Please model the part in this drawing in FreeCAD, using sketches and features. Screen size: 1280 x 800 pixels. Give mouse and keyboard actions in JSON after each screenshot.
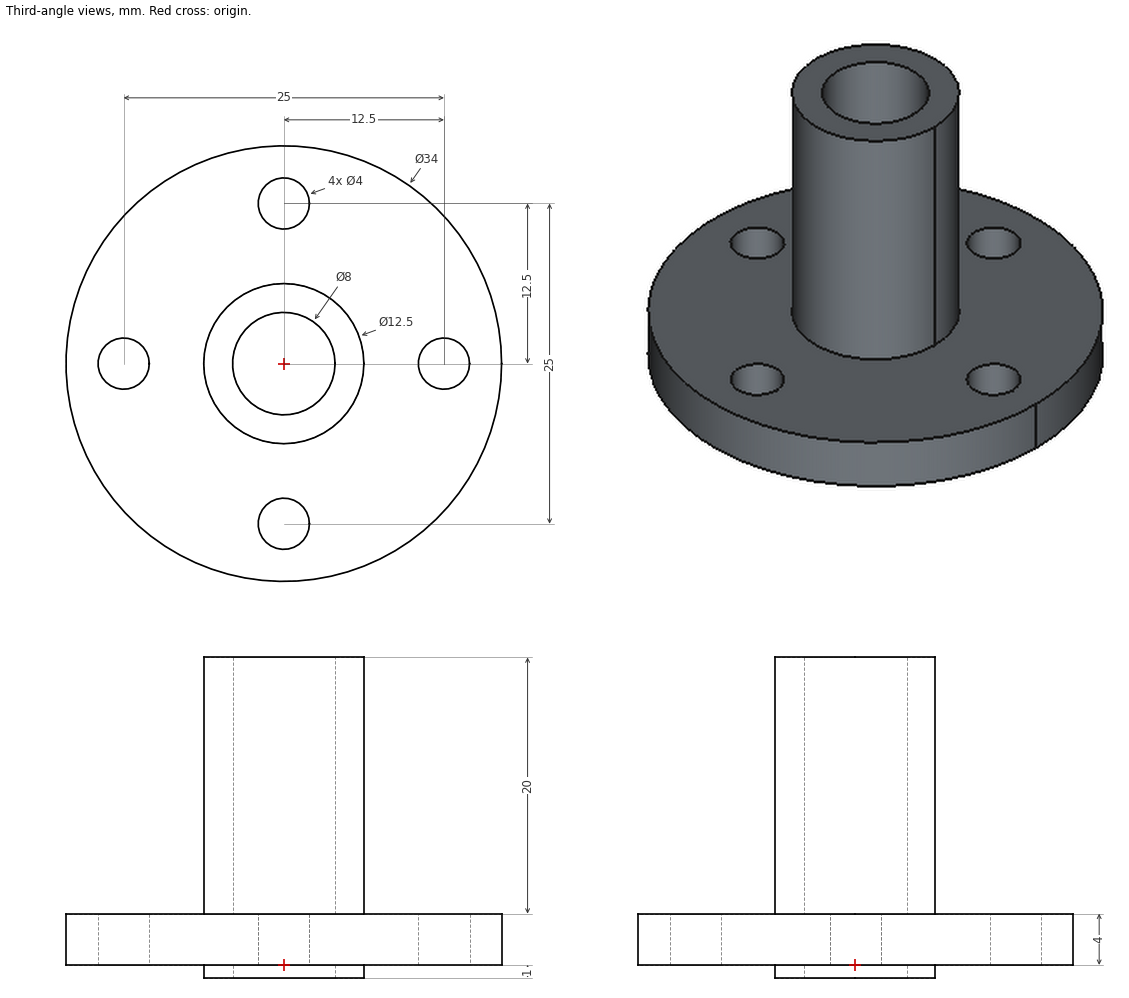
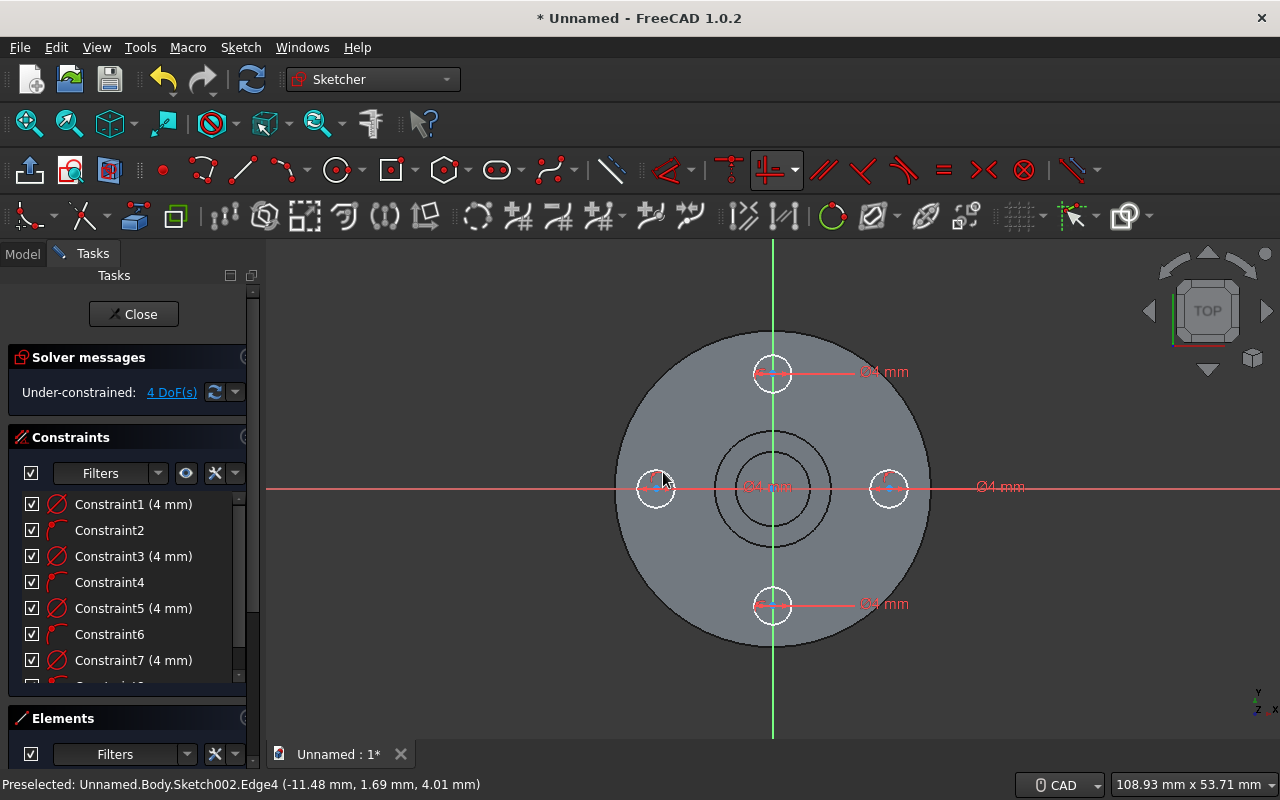
{"action": "left_click", "coordinate": [666, 170]}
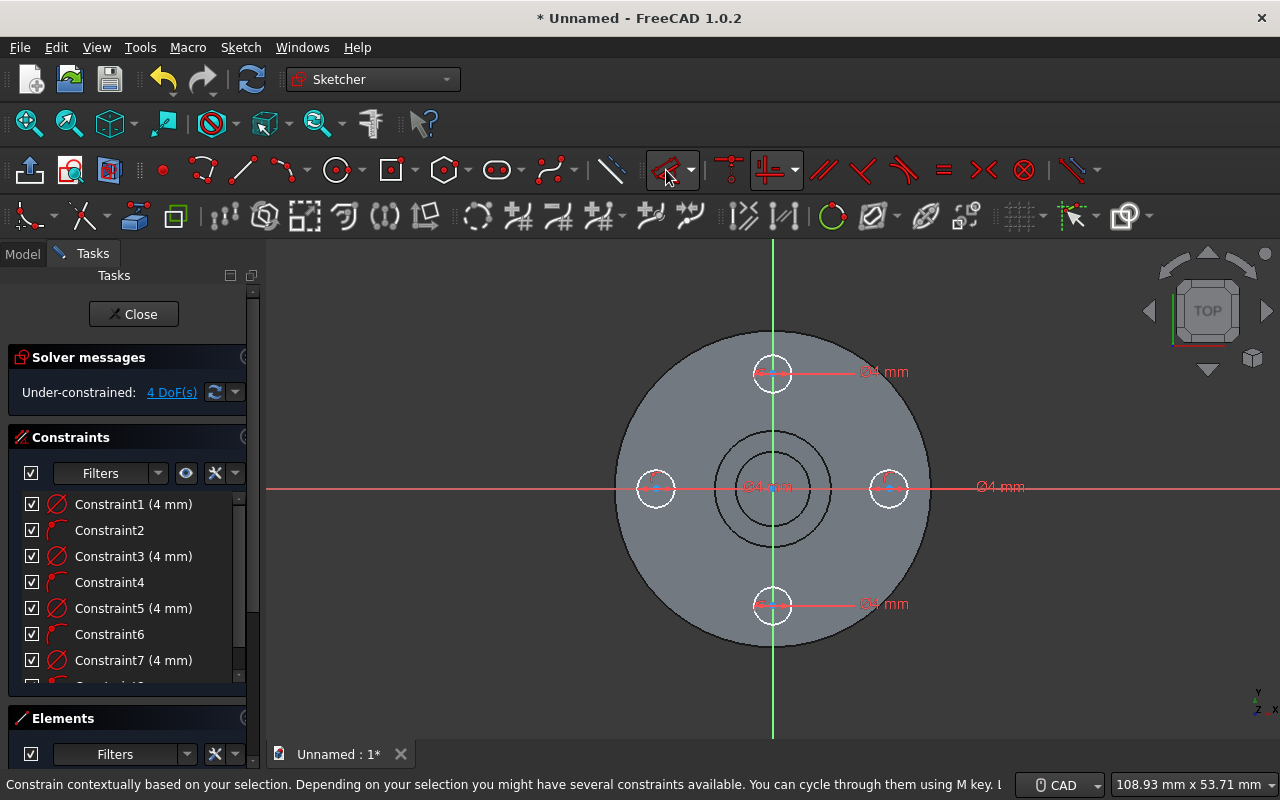
{"action": "left_click", "coordinate": [773, 374]}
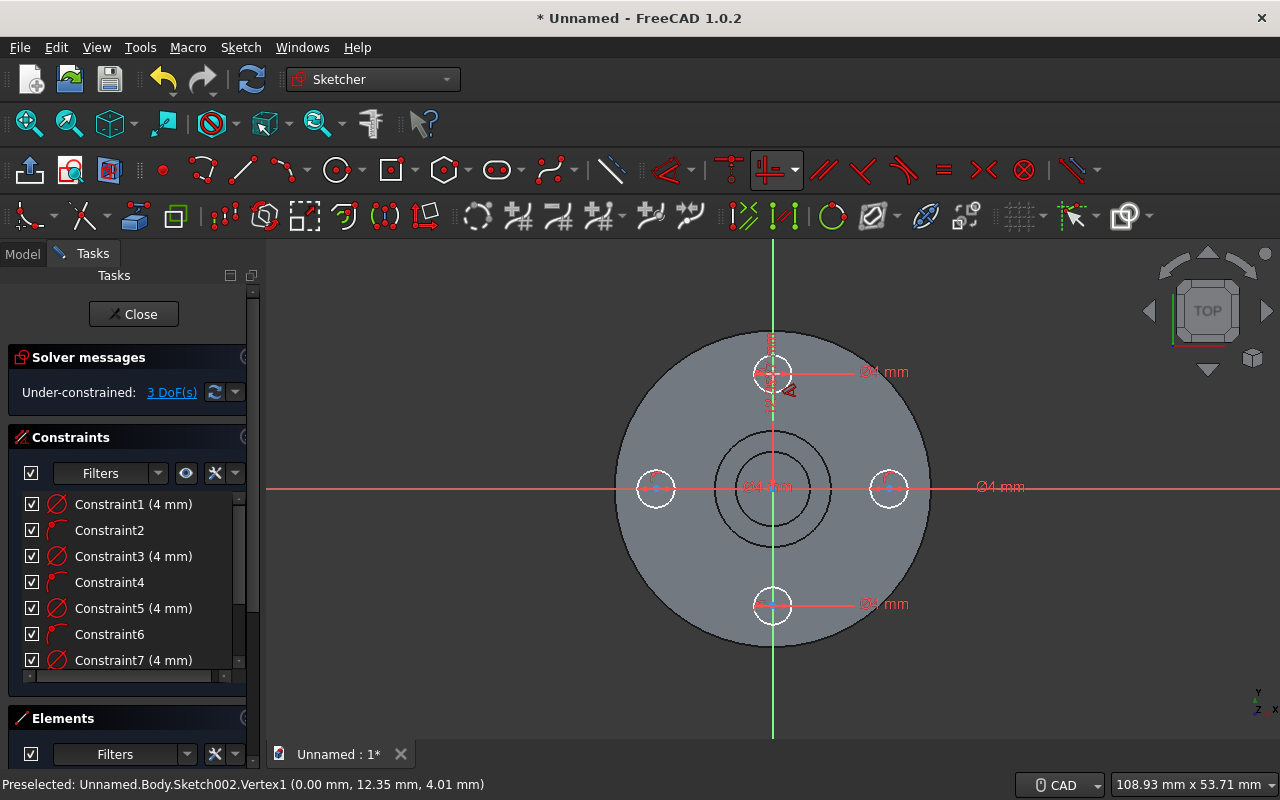
{"action": "left_click", "coordinate": [773, 606]}
{"action": "left_click", "coordinate": [807, 437]}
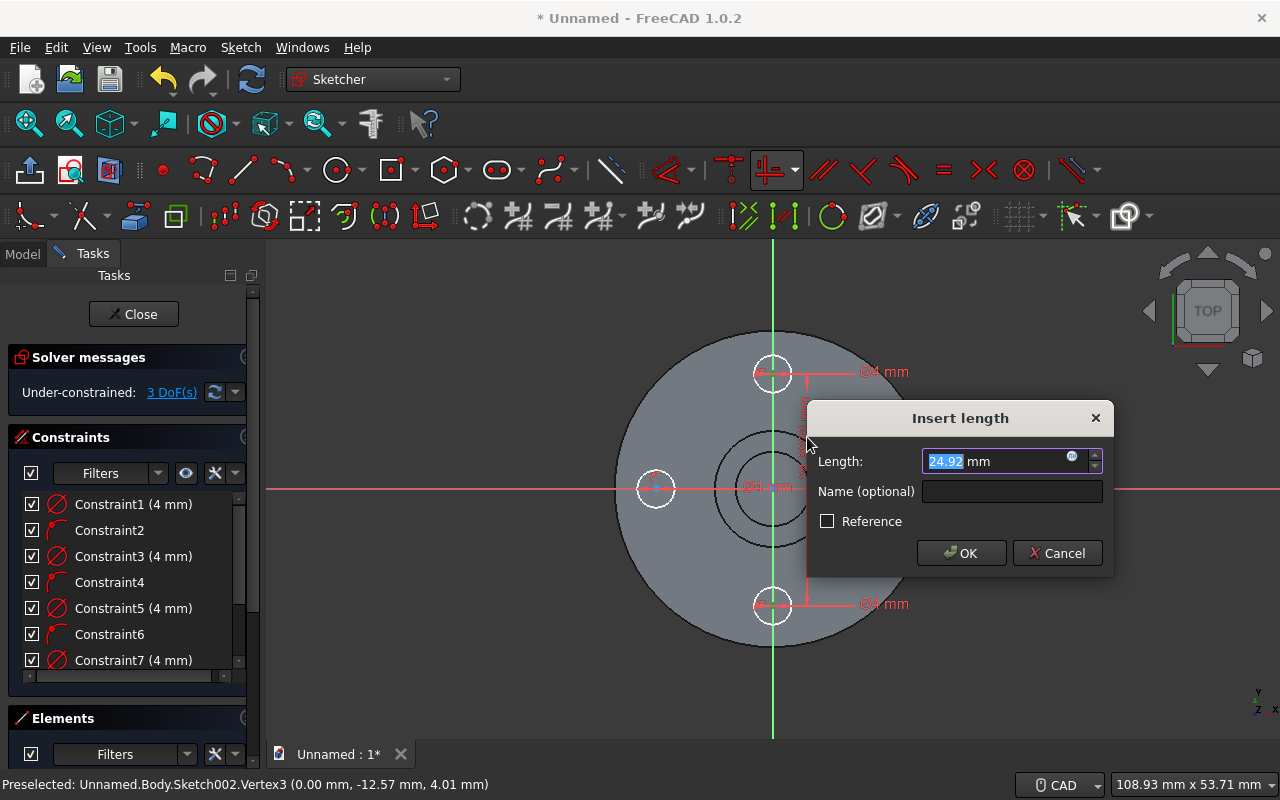
{"action": "type", "text": "25"}
{"action": "key", "text": "Return"}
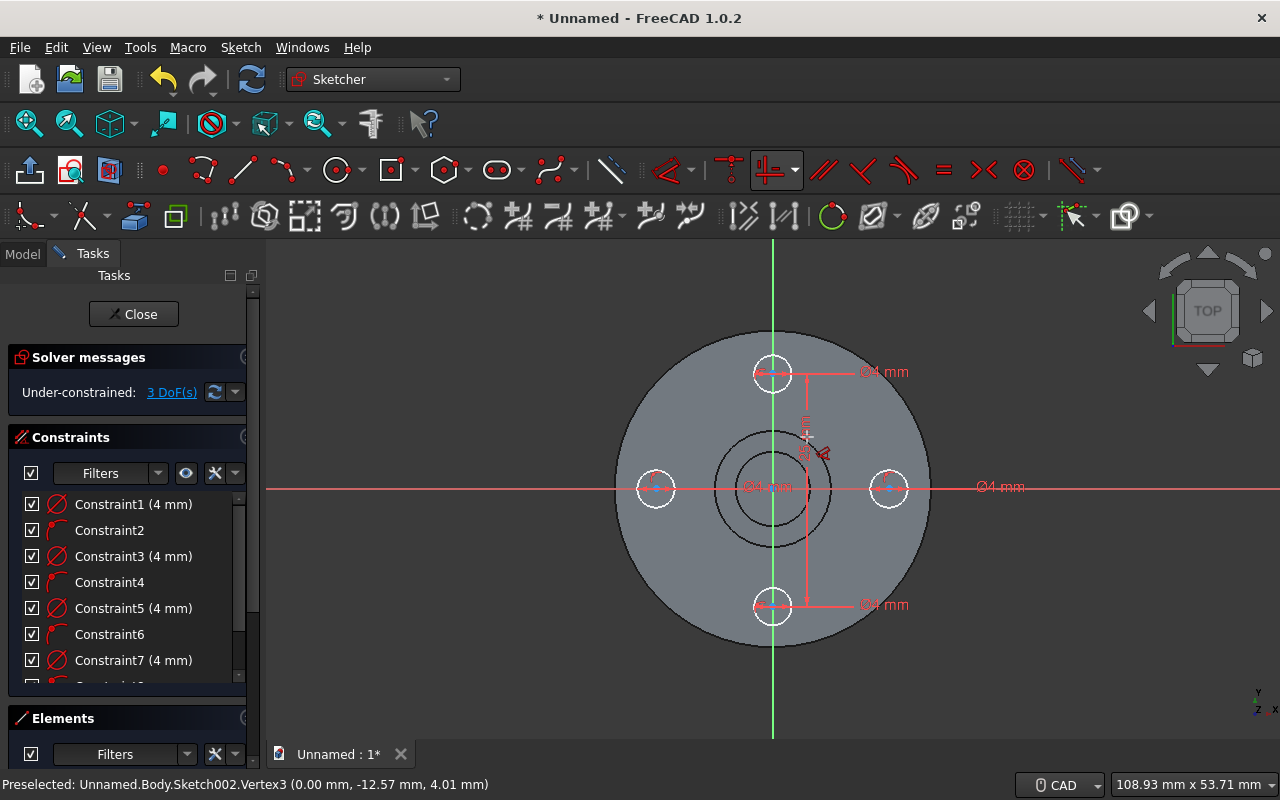
{"action": "left_click", "coordinate": [889, 489]}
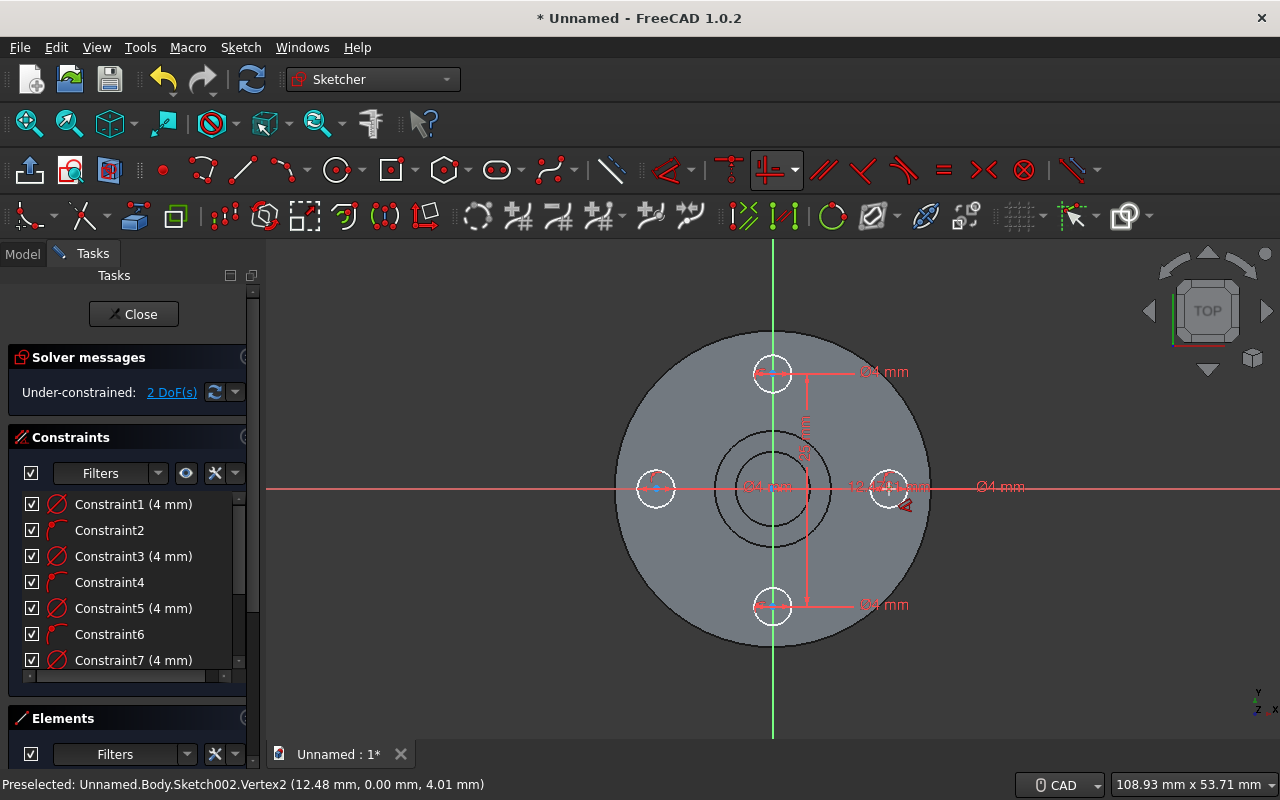
{"action": "left_click", "coordinate": [656, 489]}
{"action": "left_click", "coordinate": [719, 523]}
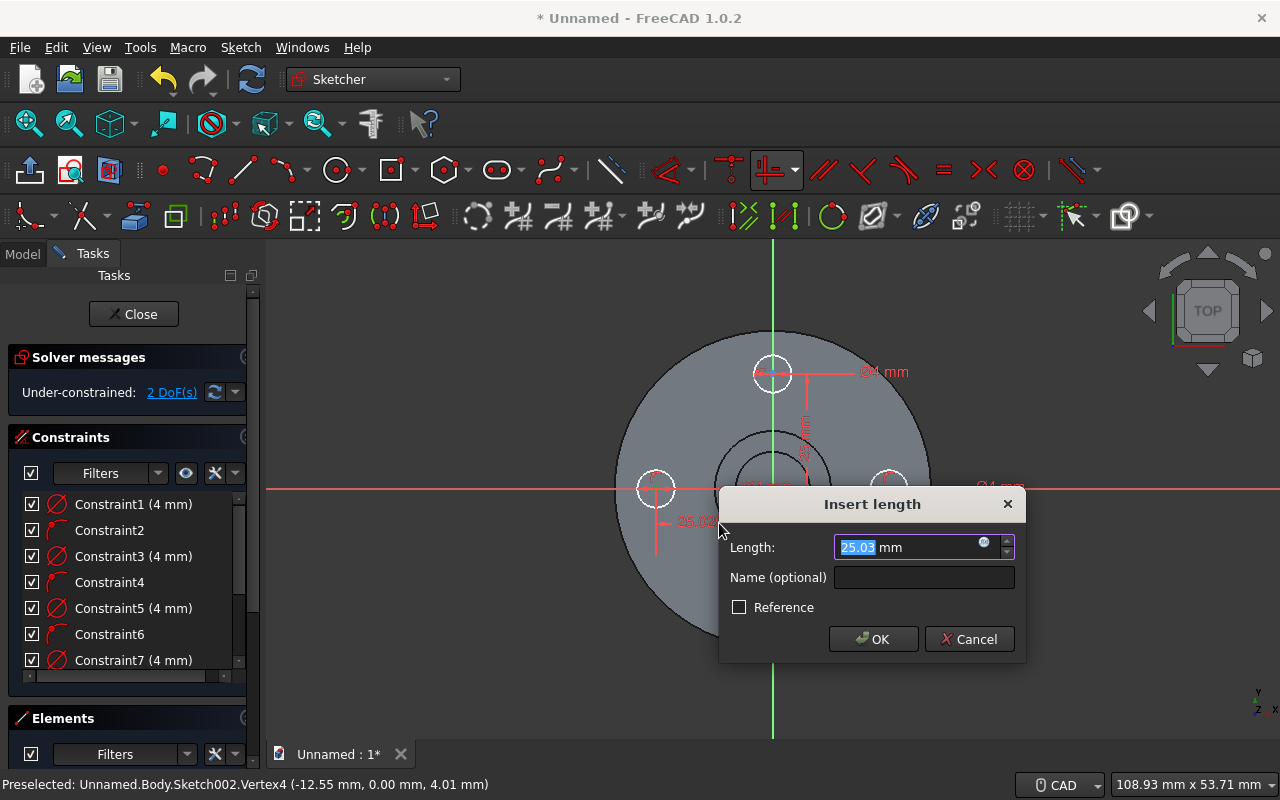
{"action": "type", "text": "25"}
{"action": "key", "text": "Return"}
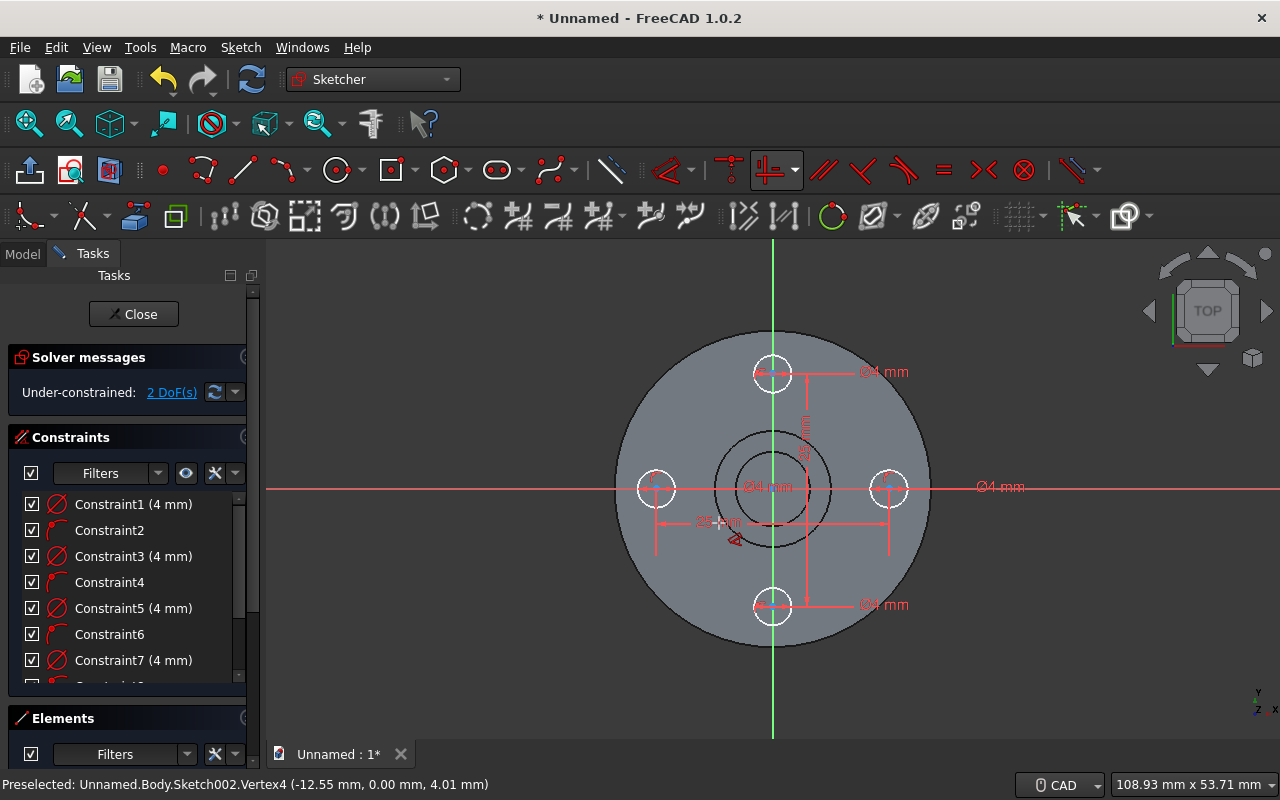
{"action": "left_click", "coordinate": [773, 374]}
{"action": "left_click", "coordinate": [807, 405]}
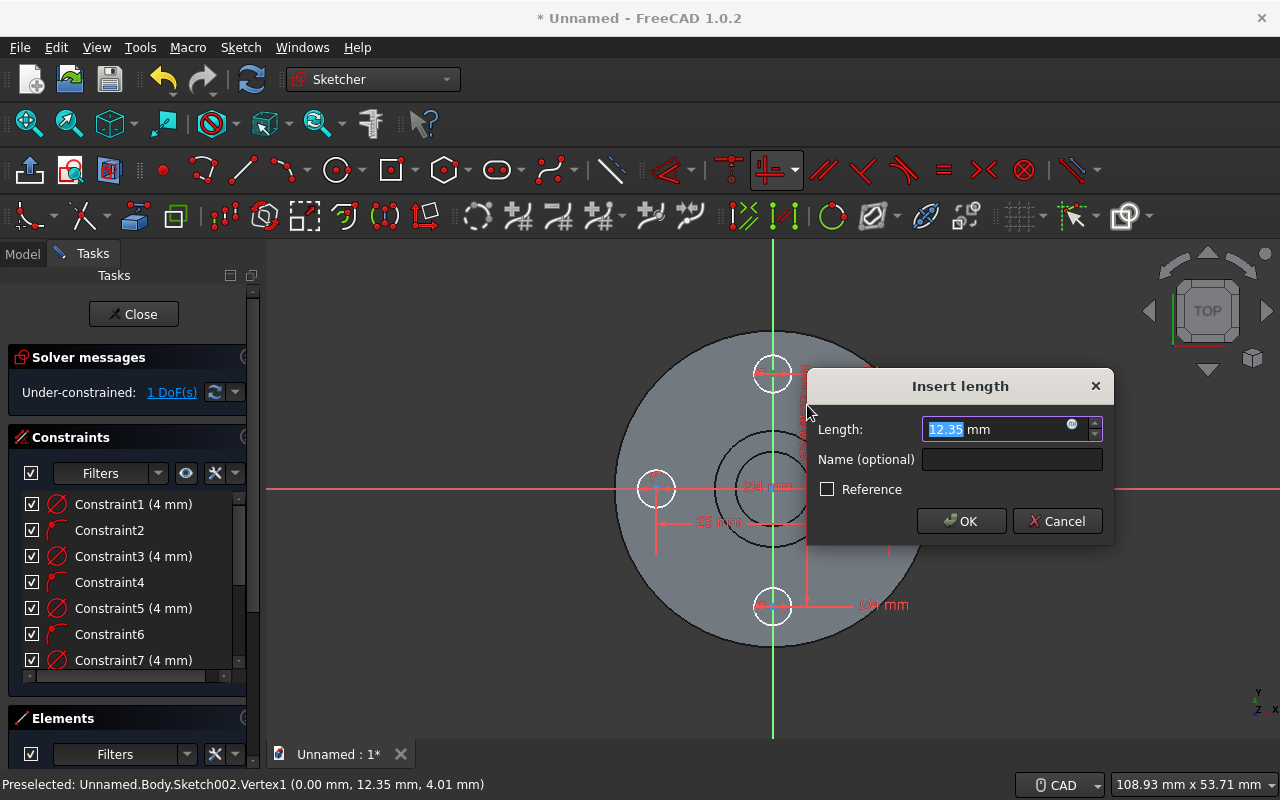
{"action": "type", "text": "12.5"}
{"action": "key", "text": "Return"}